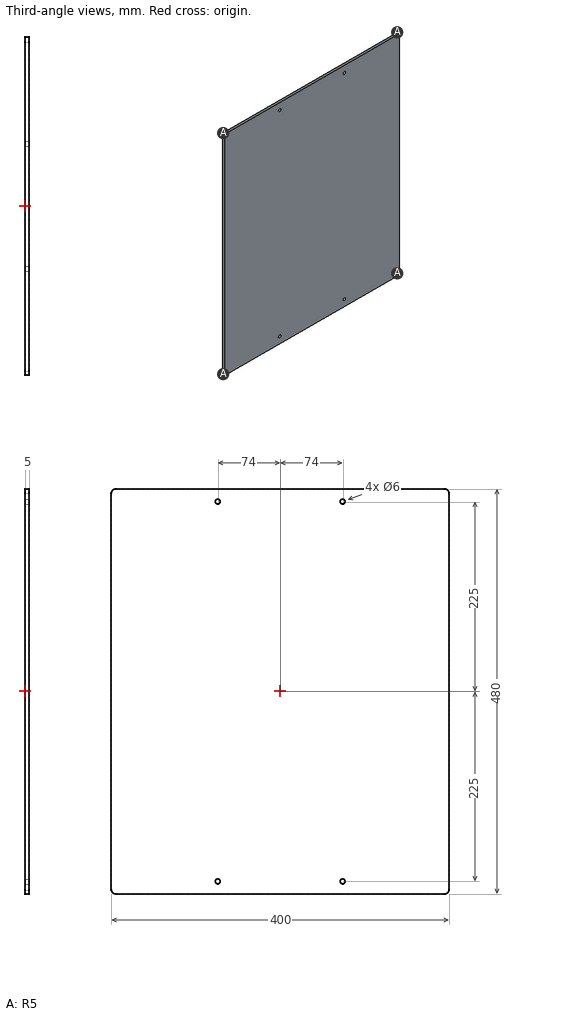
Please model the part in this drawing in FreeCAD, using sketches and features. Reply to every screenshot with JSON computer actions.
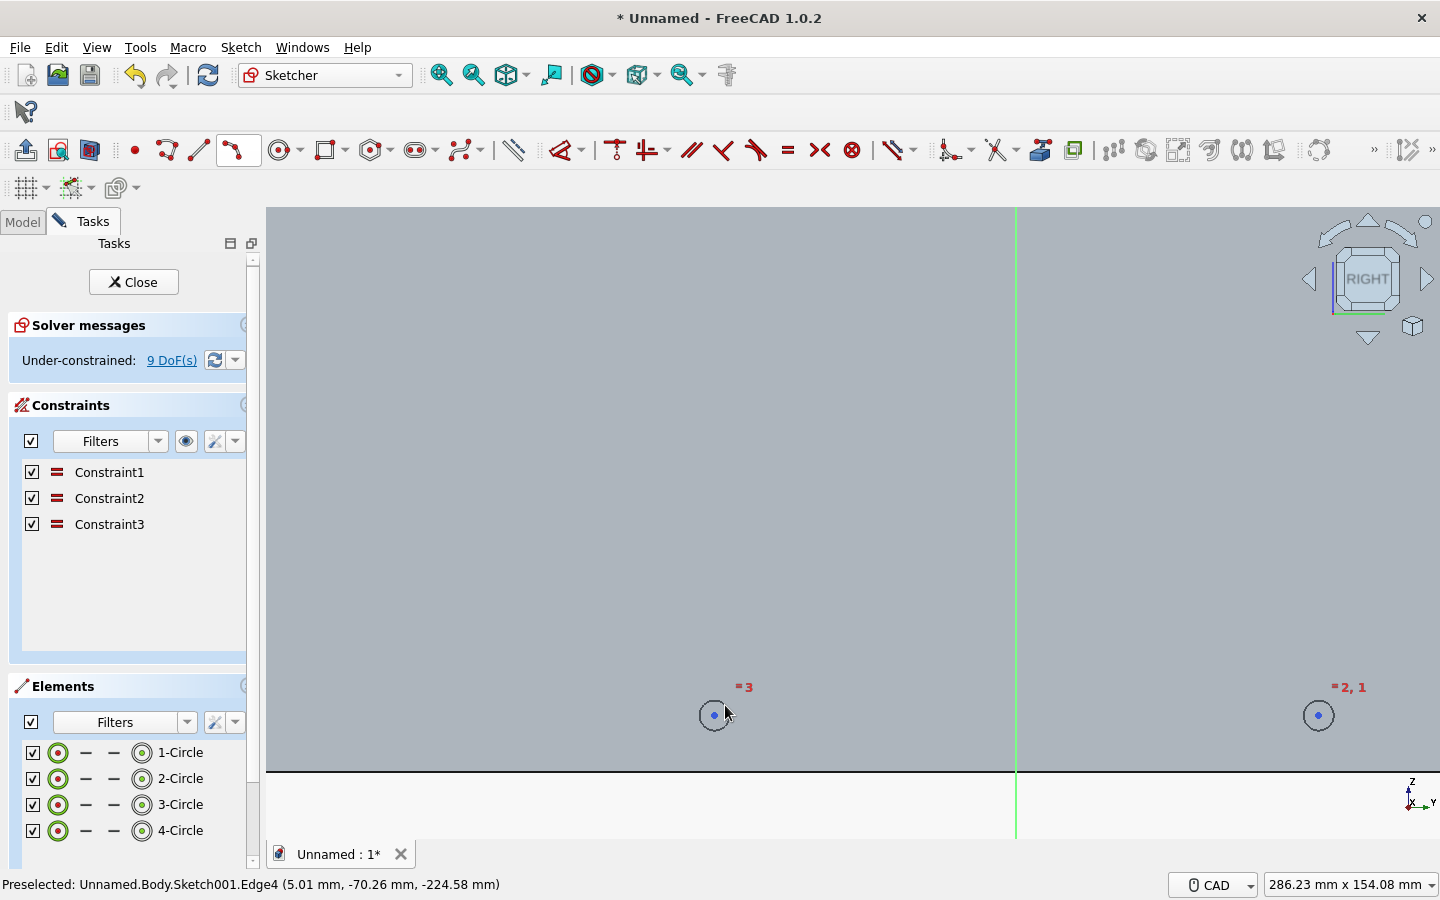
{"action": "scroll", "coordinate": [726, 709], "scroll_direction": "down", "scroll_amount": 8}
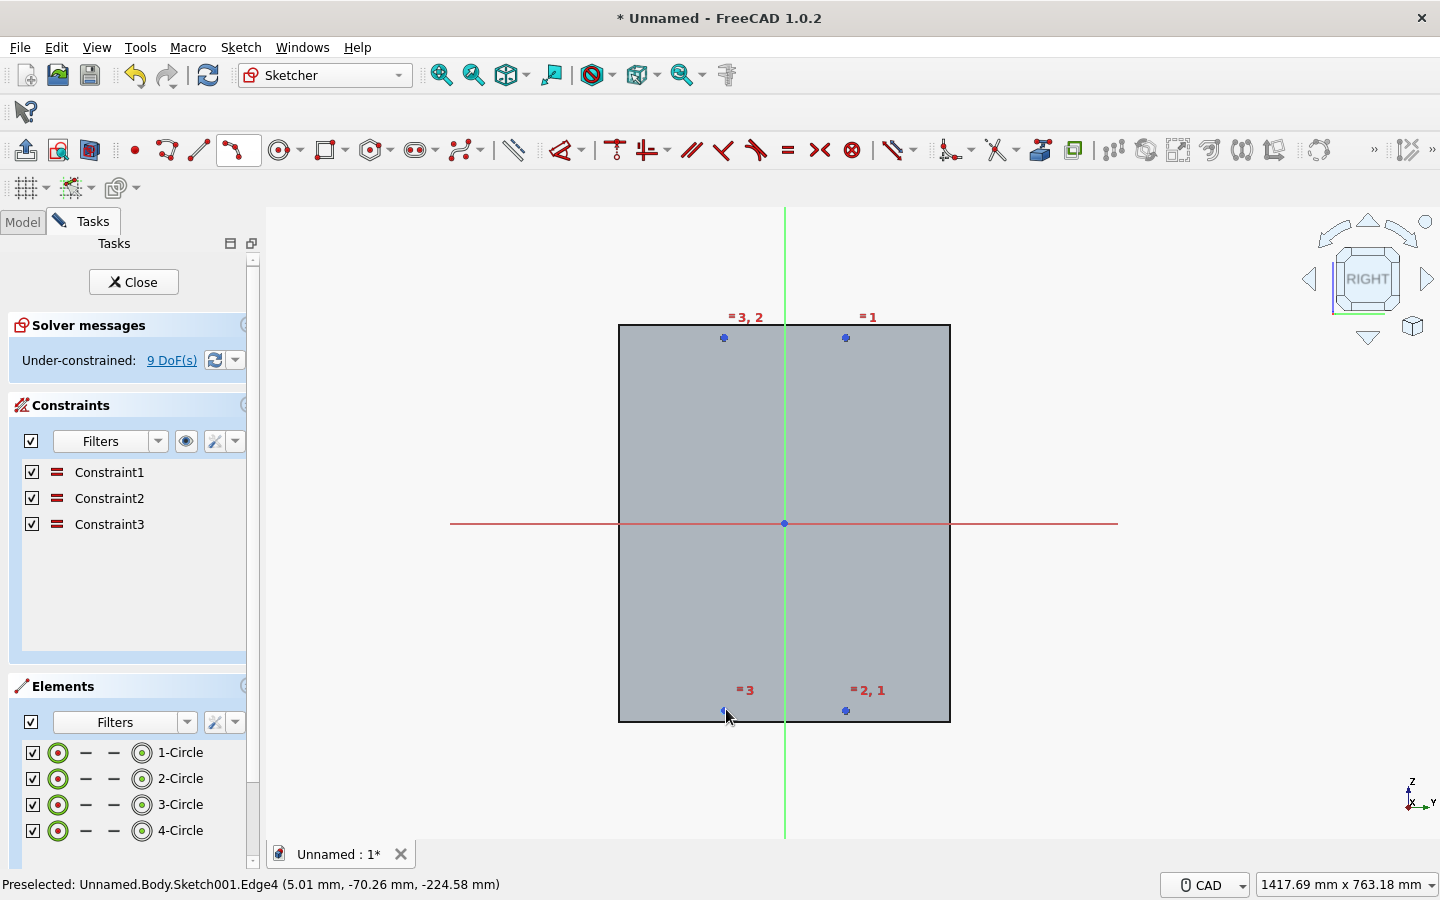
{"action": "left_click", "coordinate": [846, 338]}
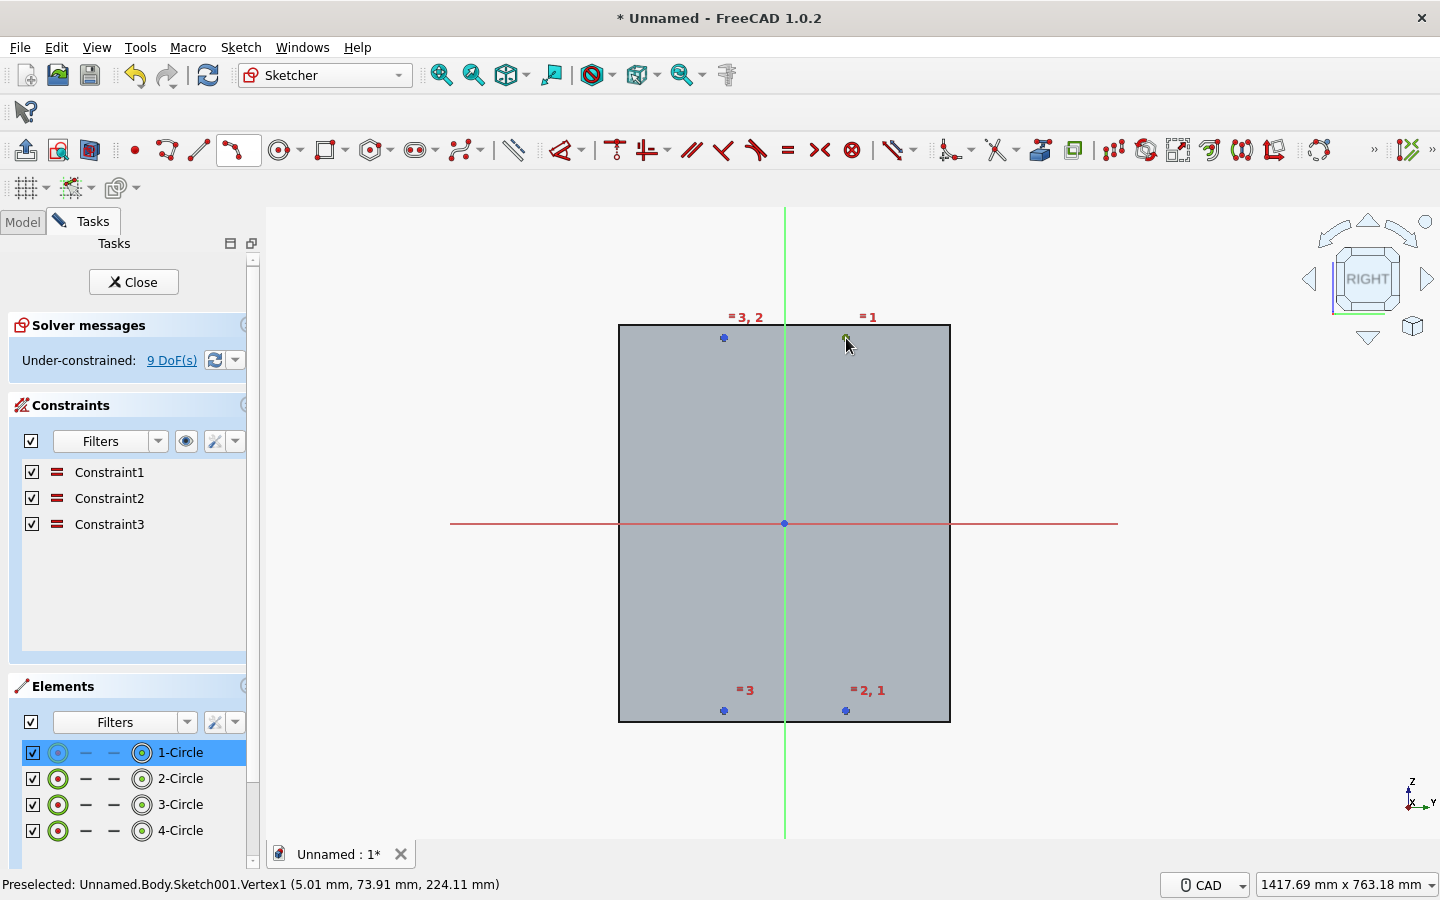
{"action": "left_click", "coordinate": [846, 711]}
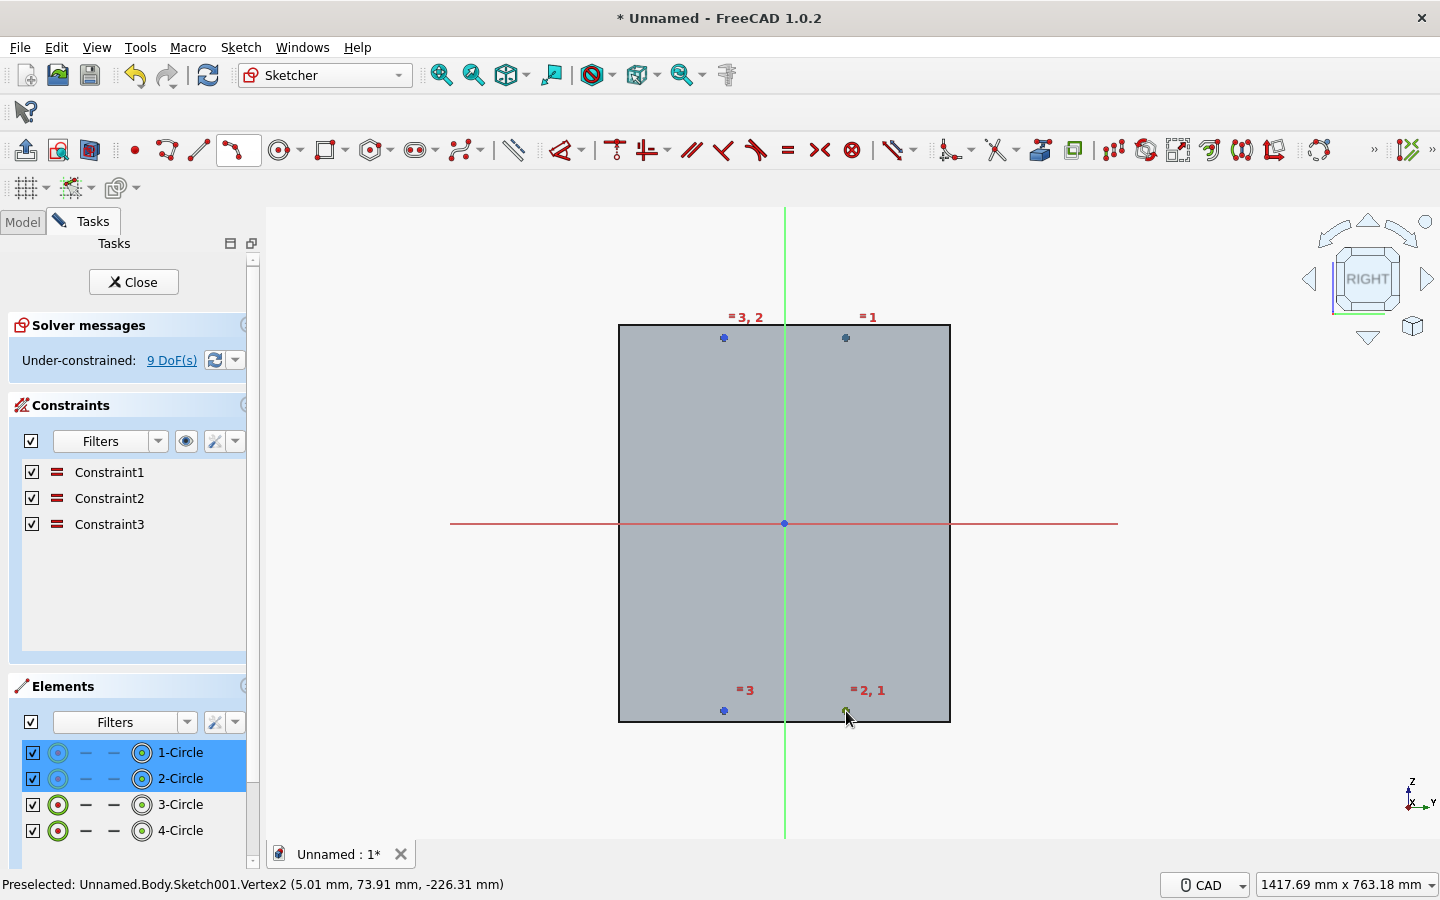
{"action": "key", "text": "v"}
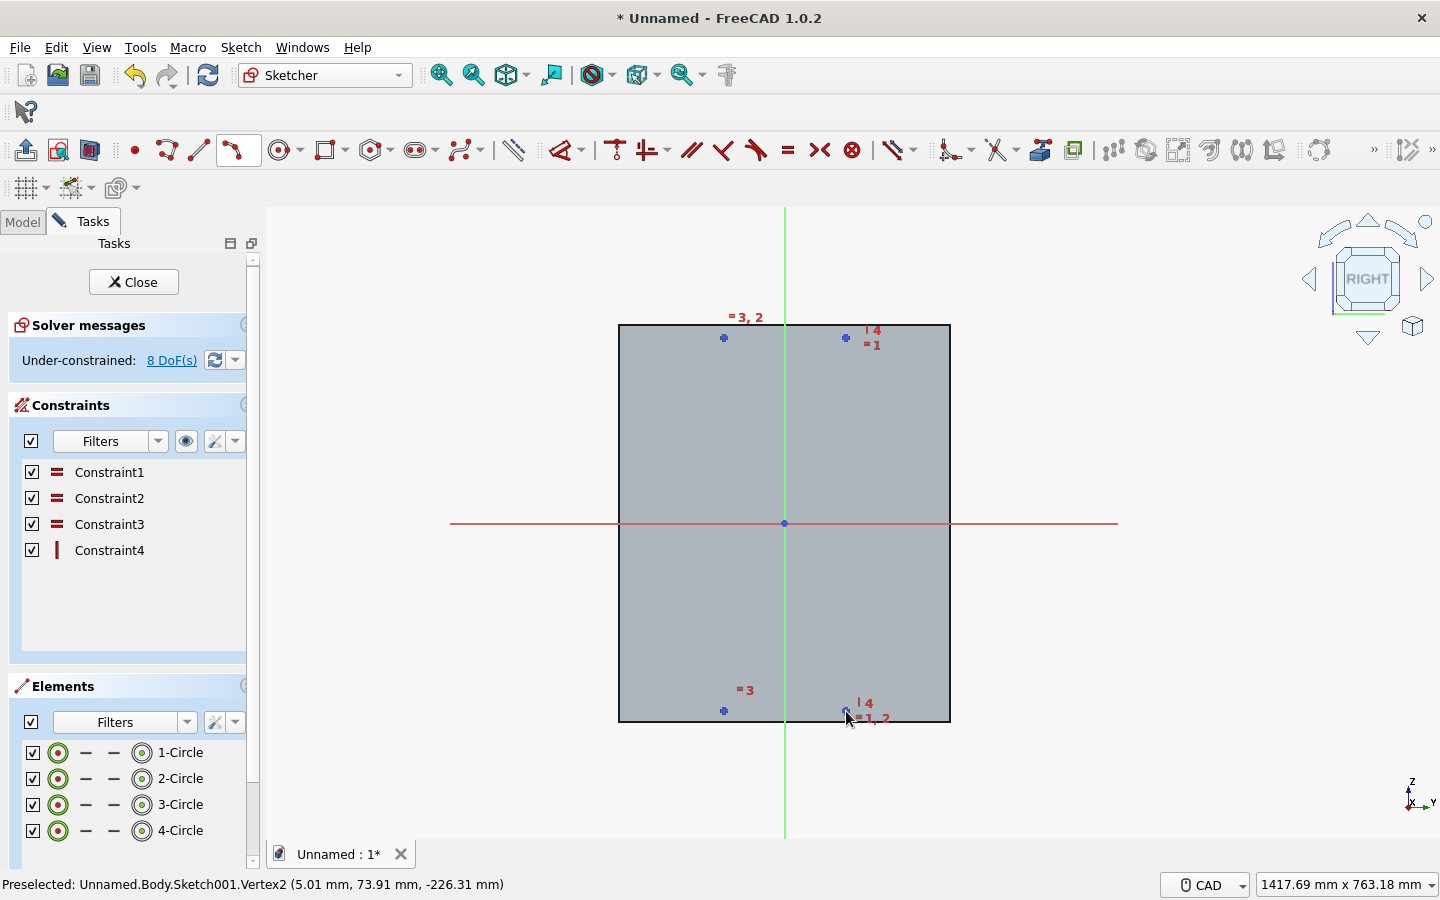
{"action": "left_click", "coordinate": [846, 338]}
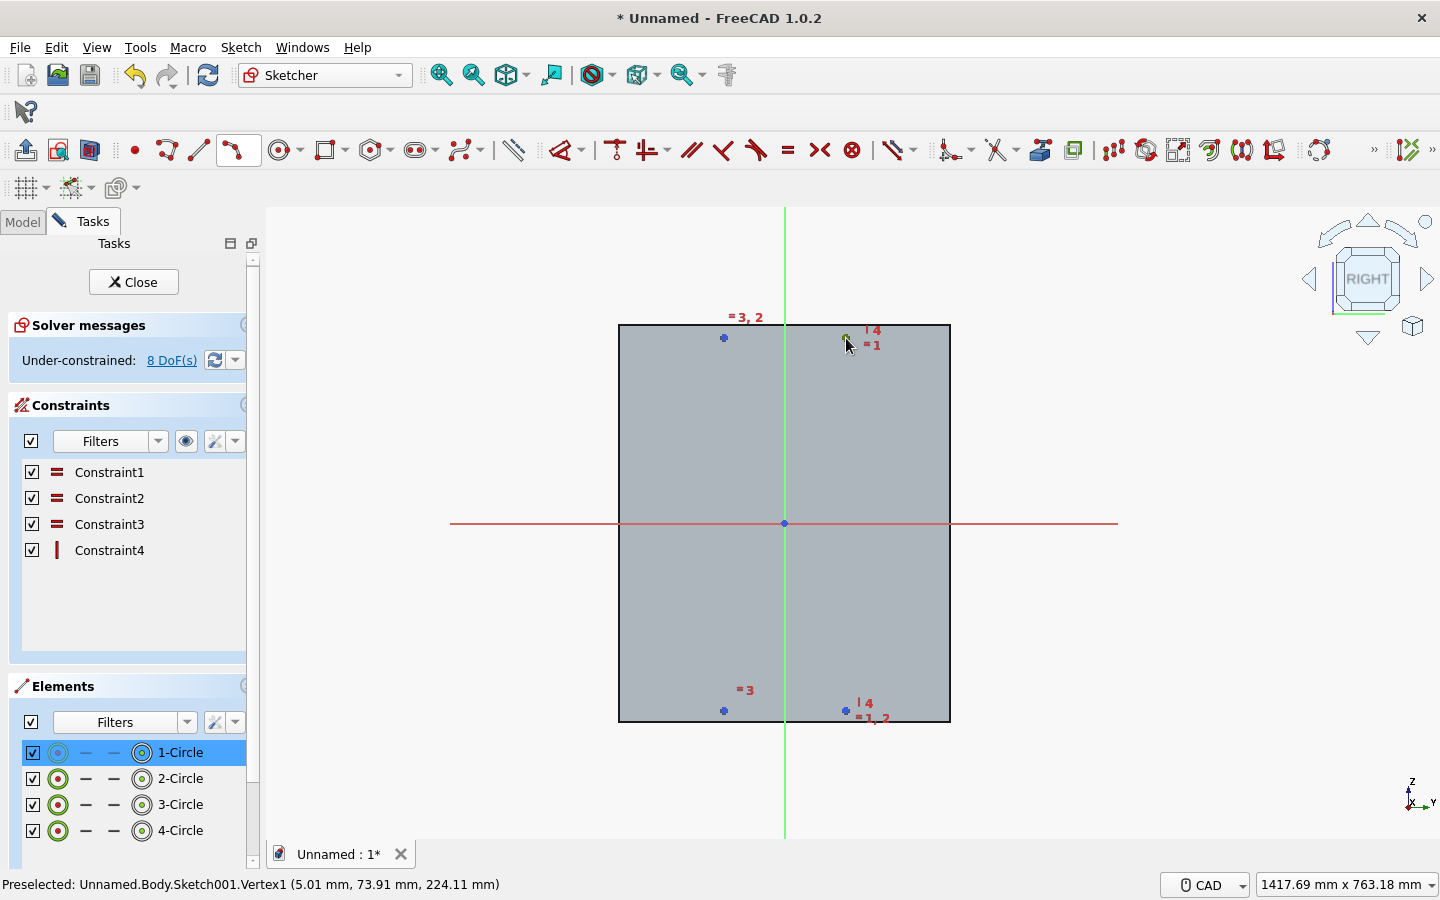
{"action": "left_click", "coordinate": [724, 338]}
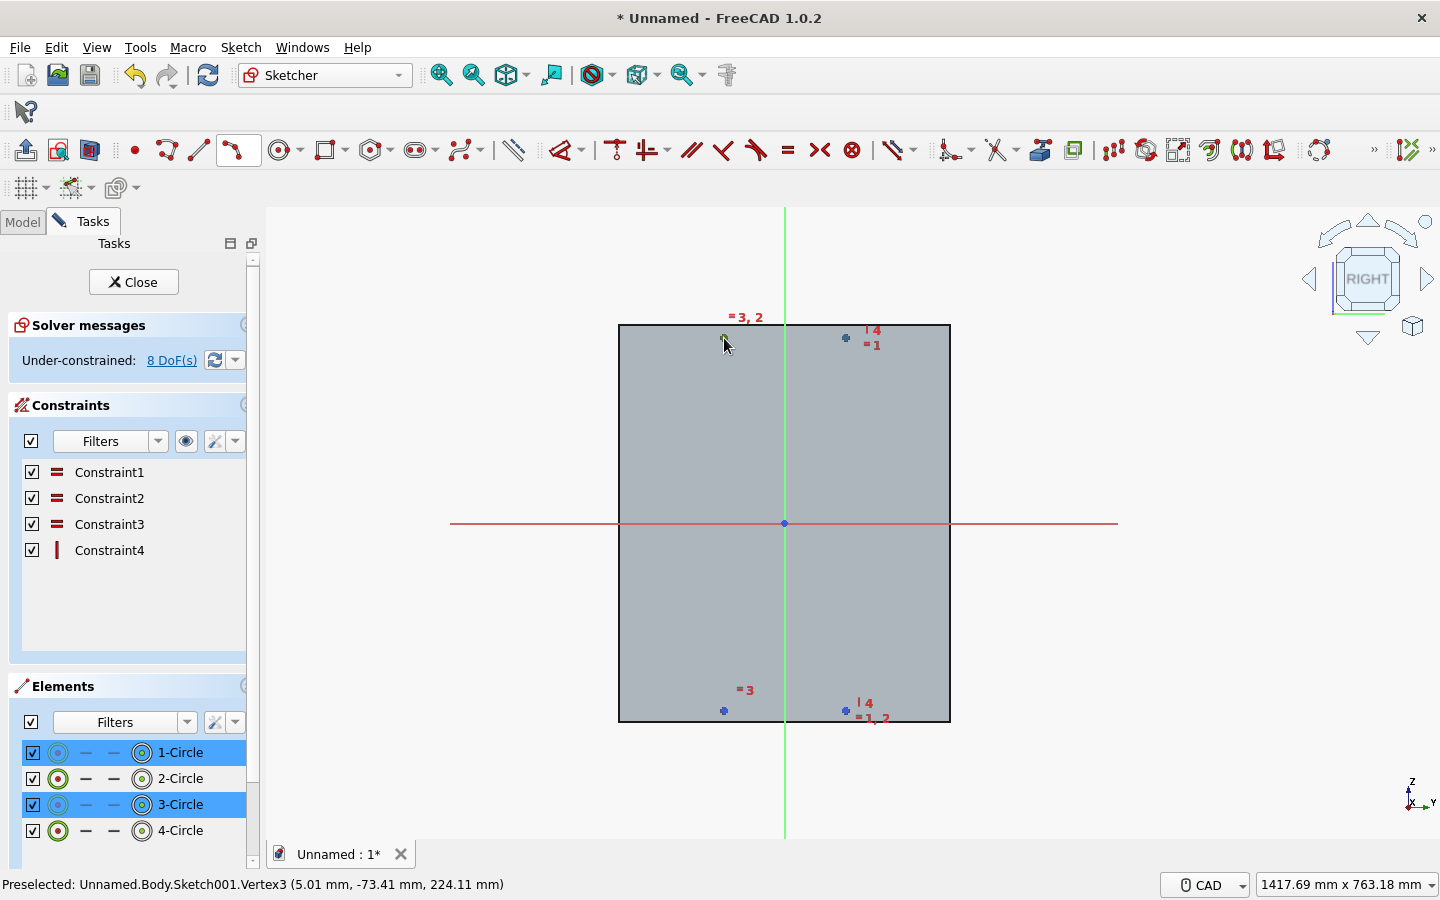
{"action": "key", "text": "h"}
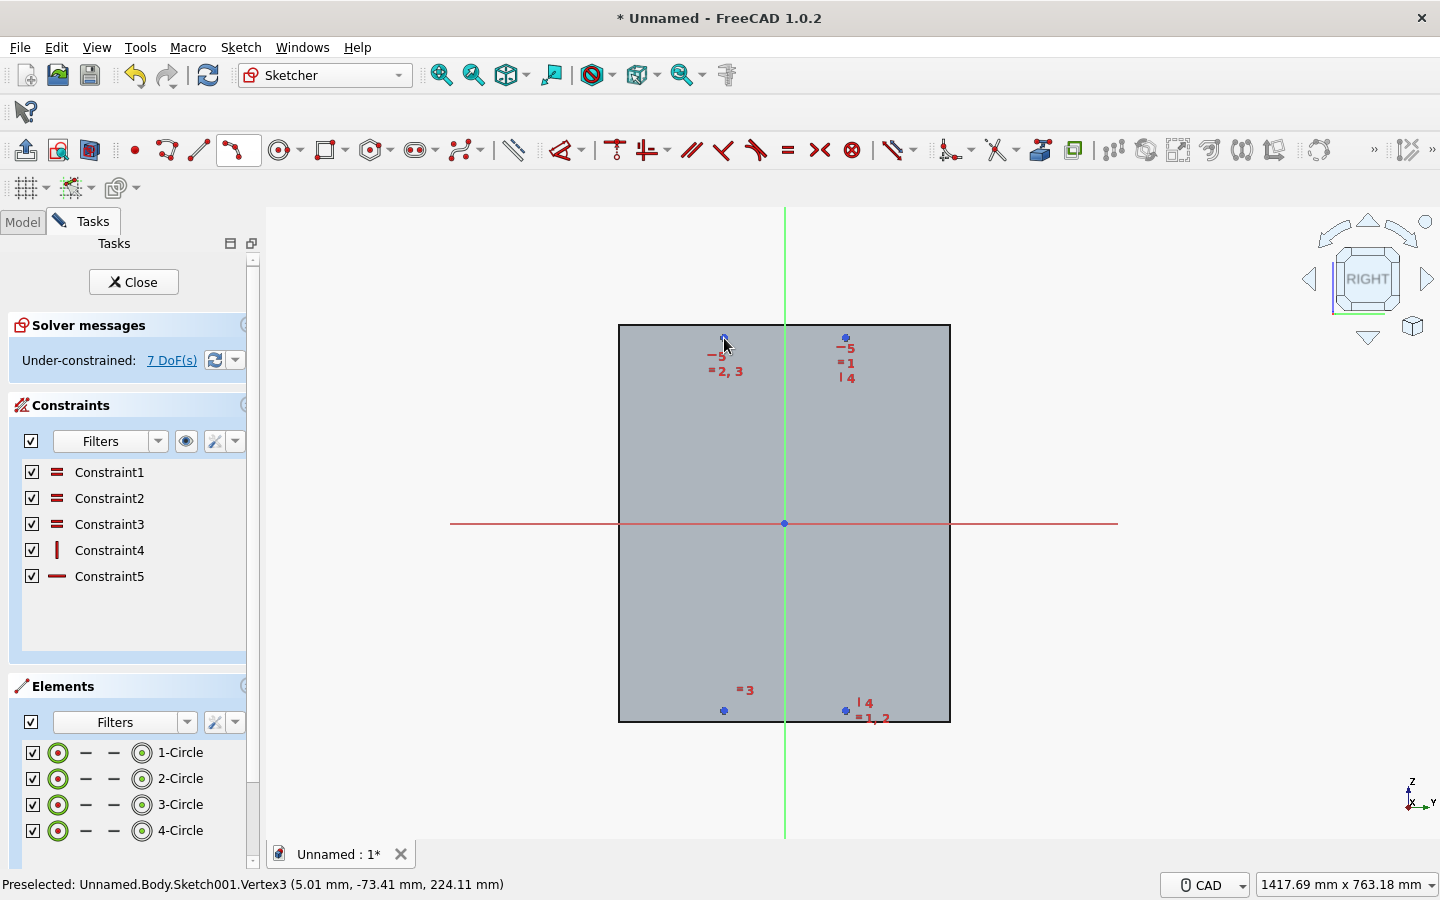
{"action": "left_click", "coordinate": [724, 338]}